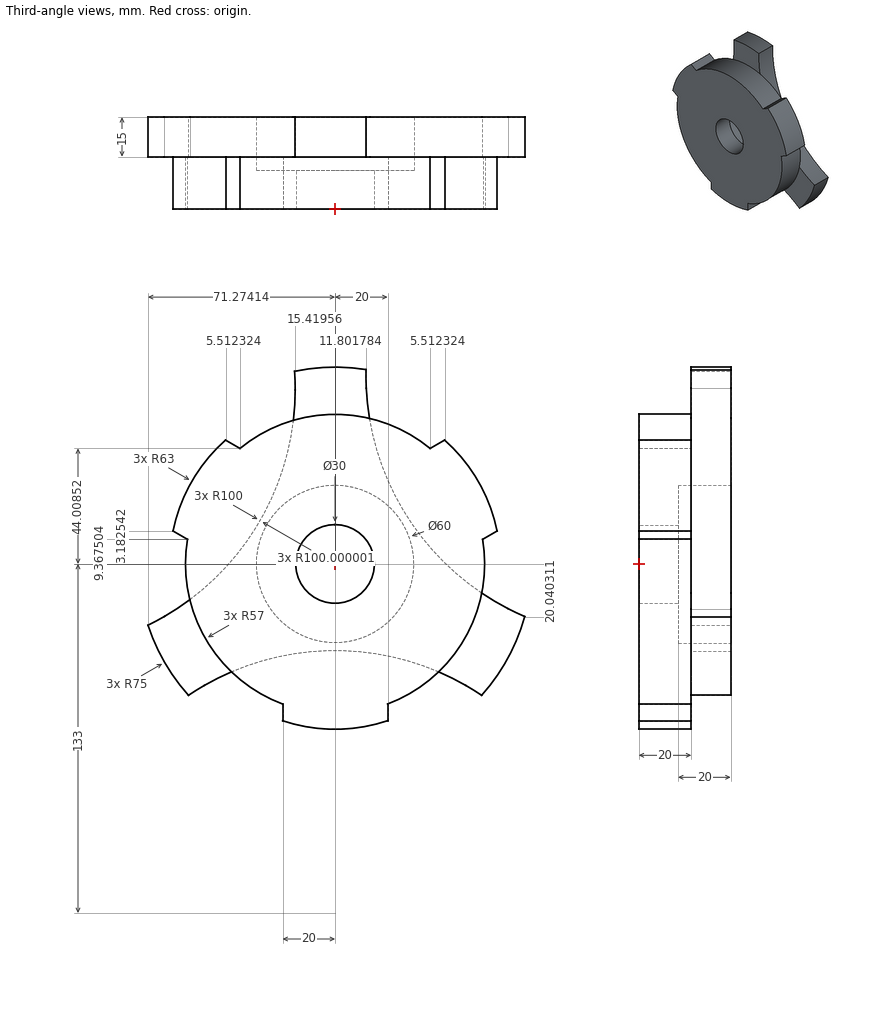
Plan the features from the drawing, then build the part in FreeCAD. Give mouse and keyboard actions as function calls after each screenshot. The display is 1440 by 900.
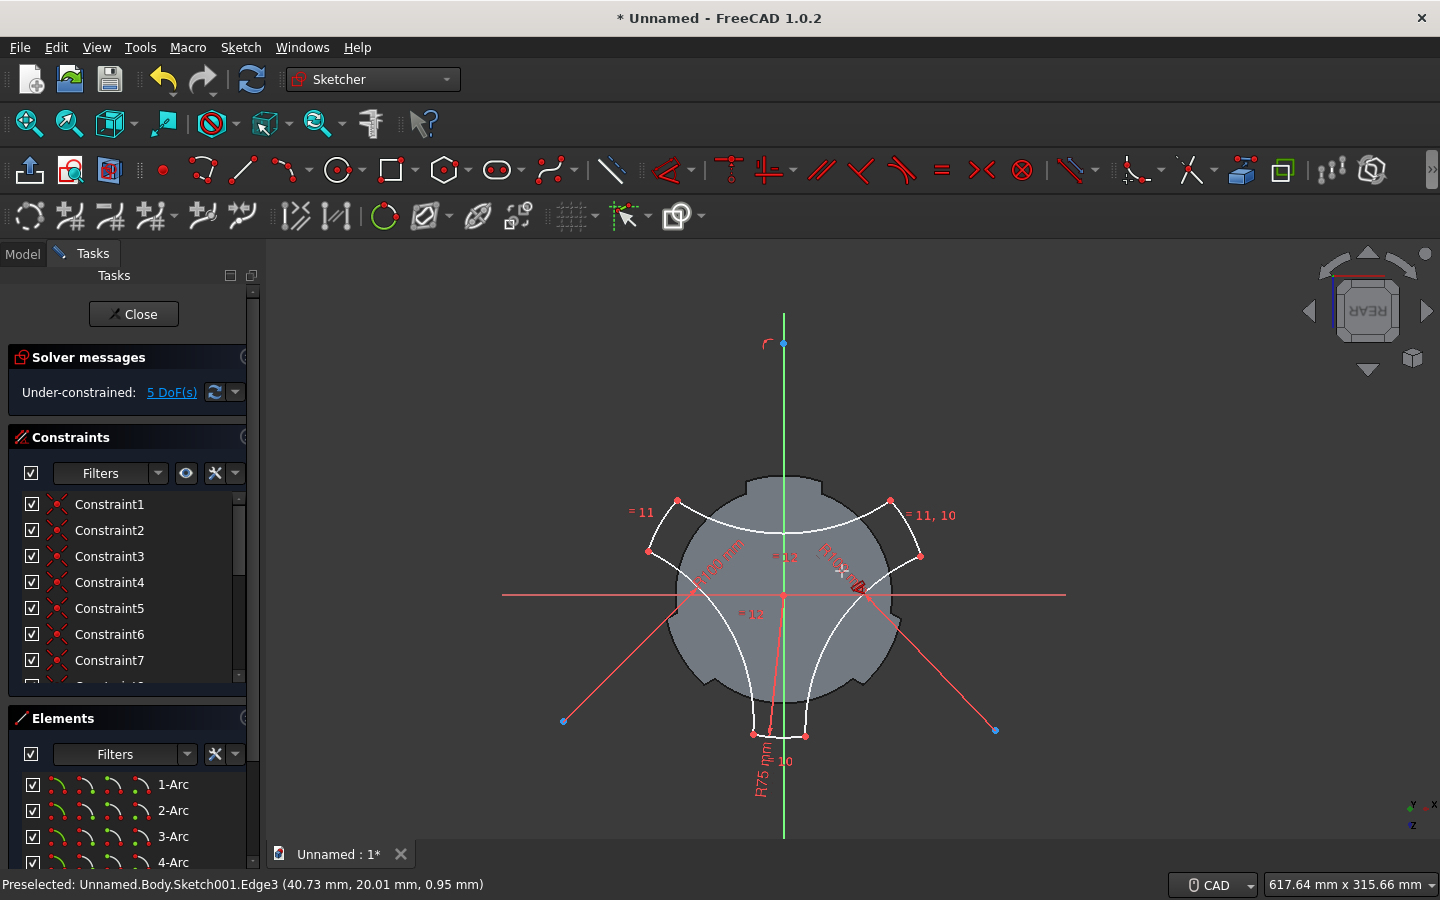
click(784, 343)
click(750, 469)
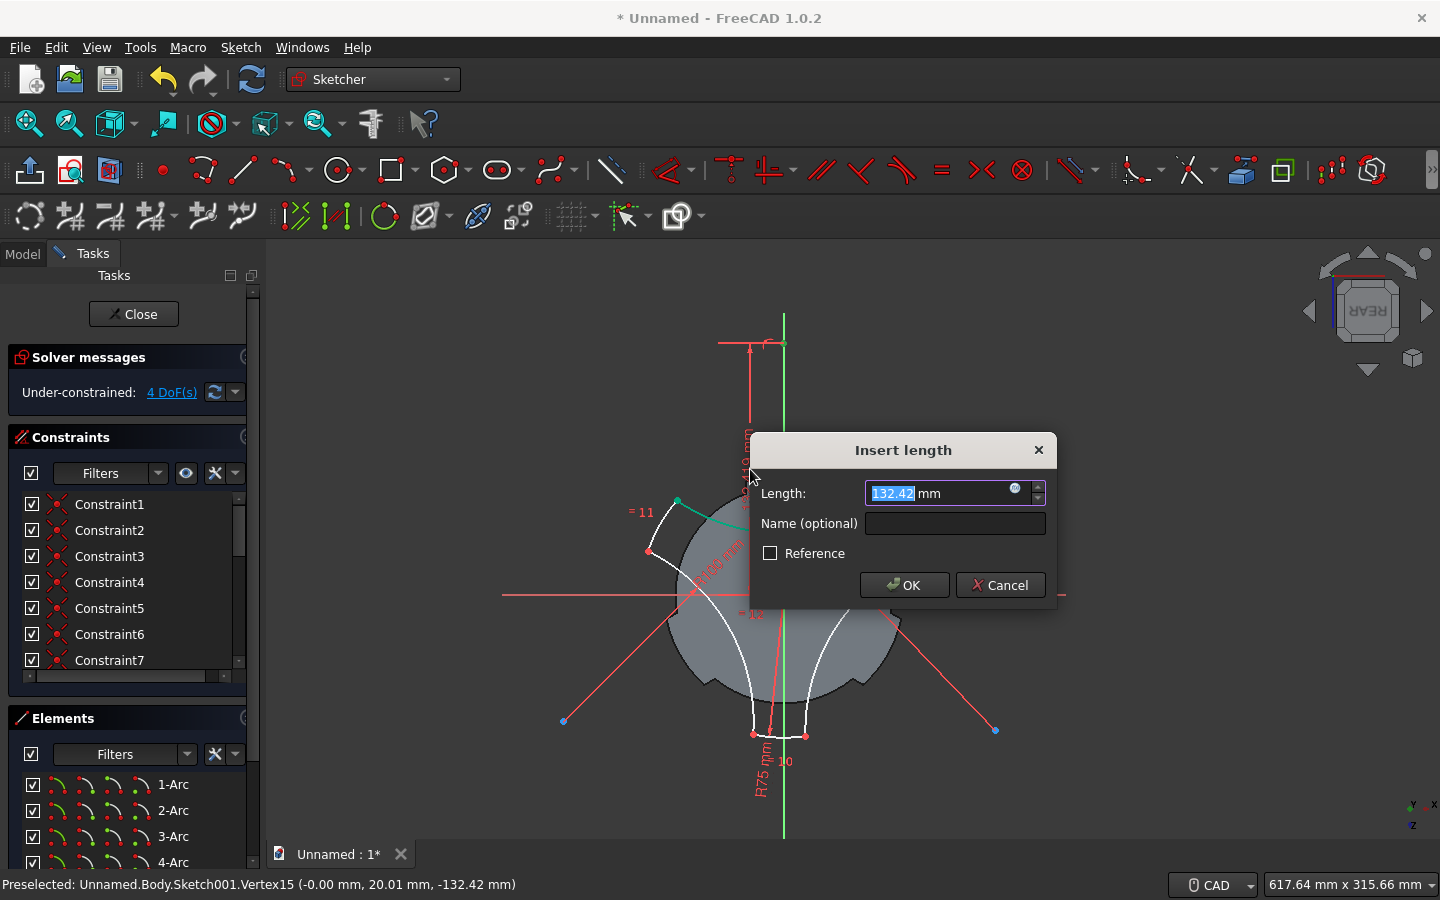
text(133)
key(Return)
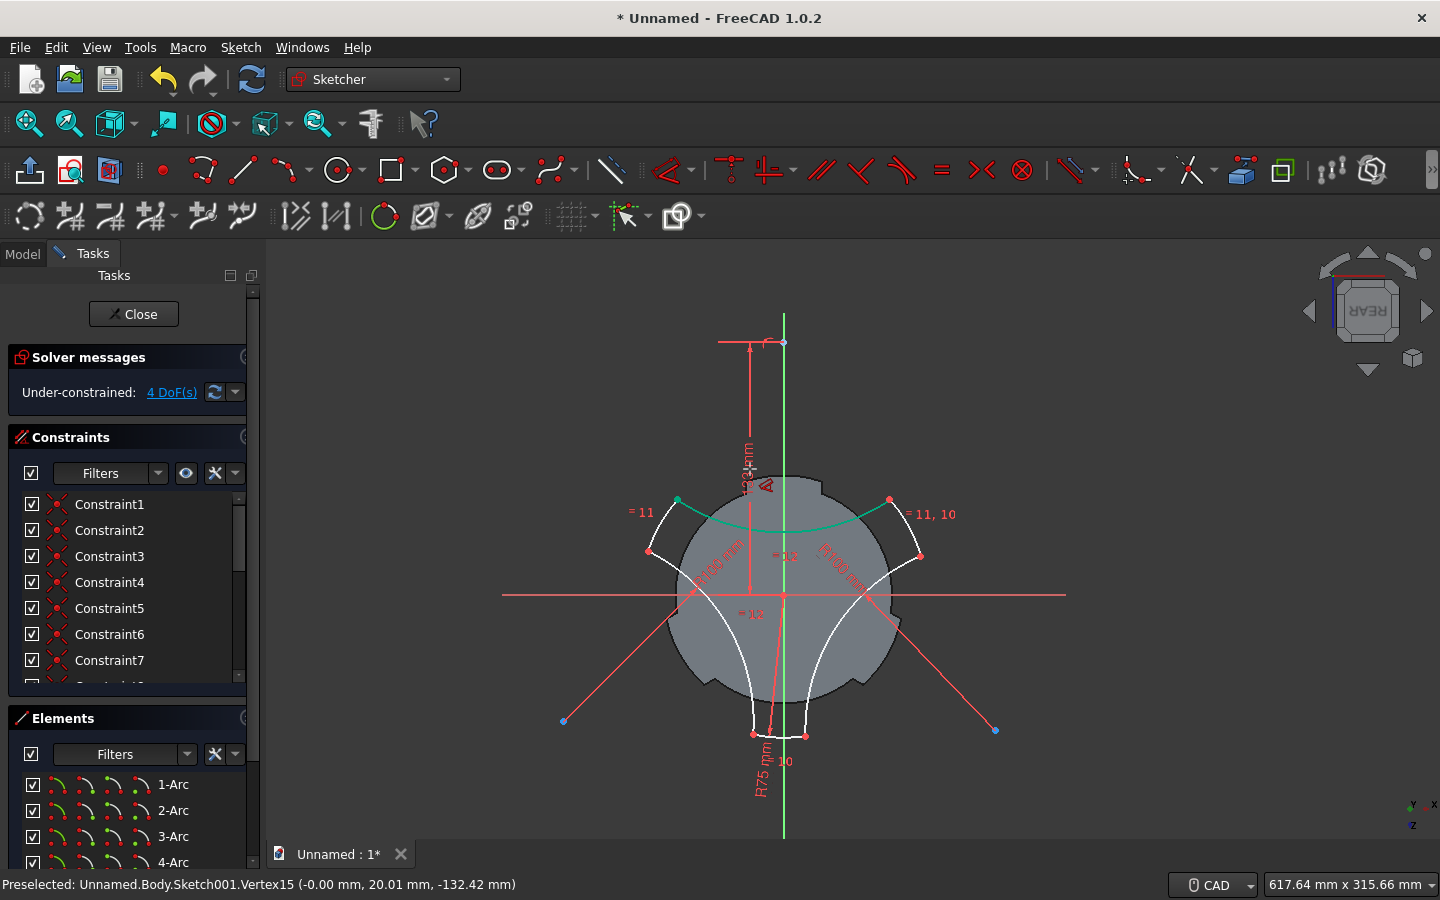
scroll(753, 734, up, 2)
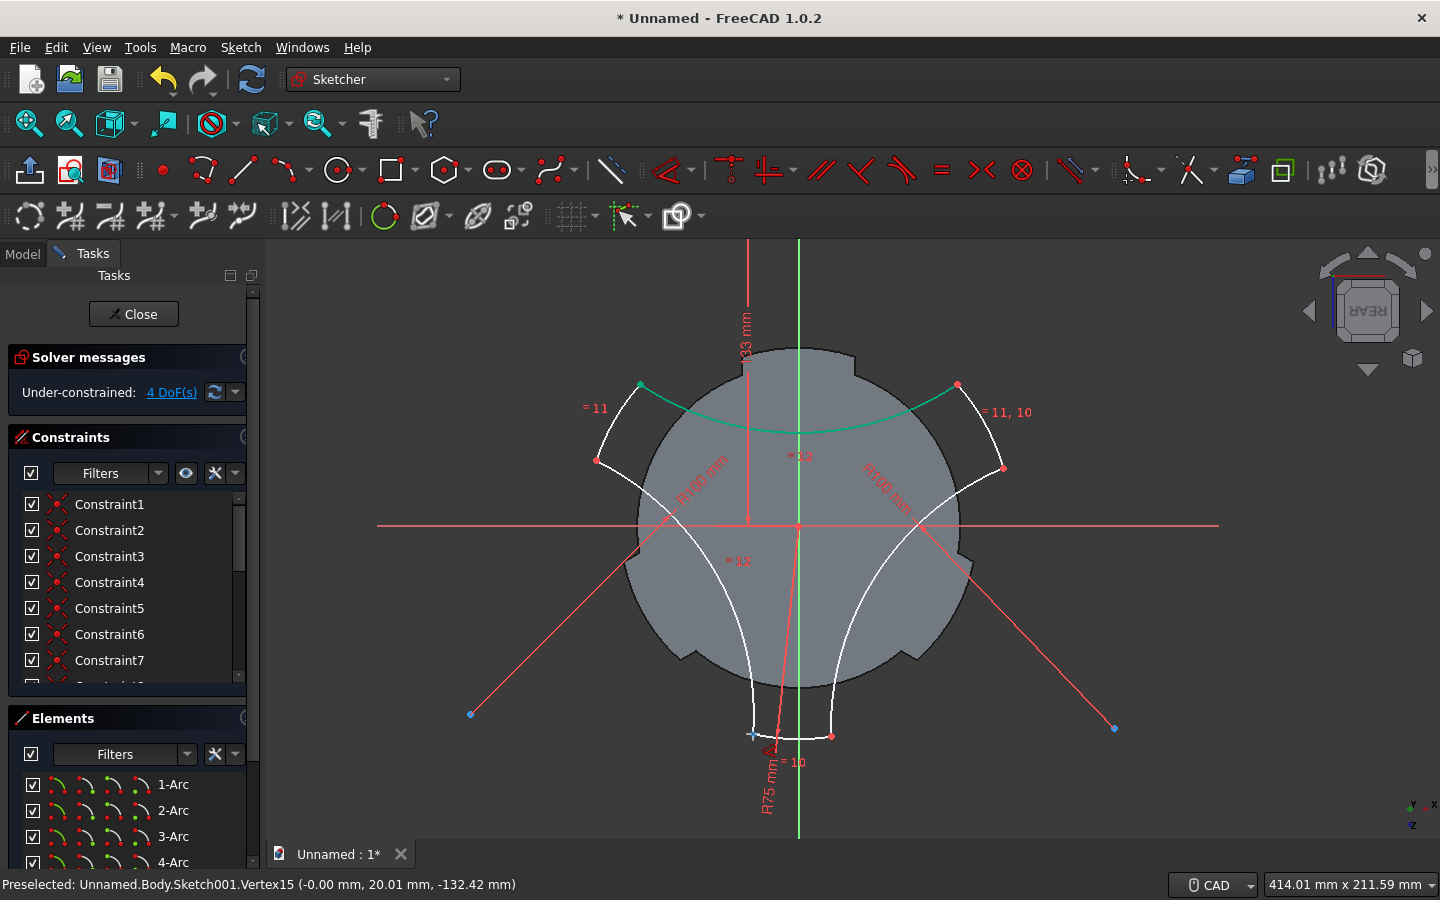
click(753, 734)
click(776, 492)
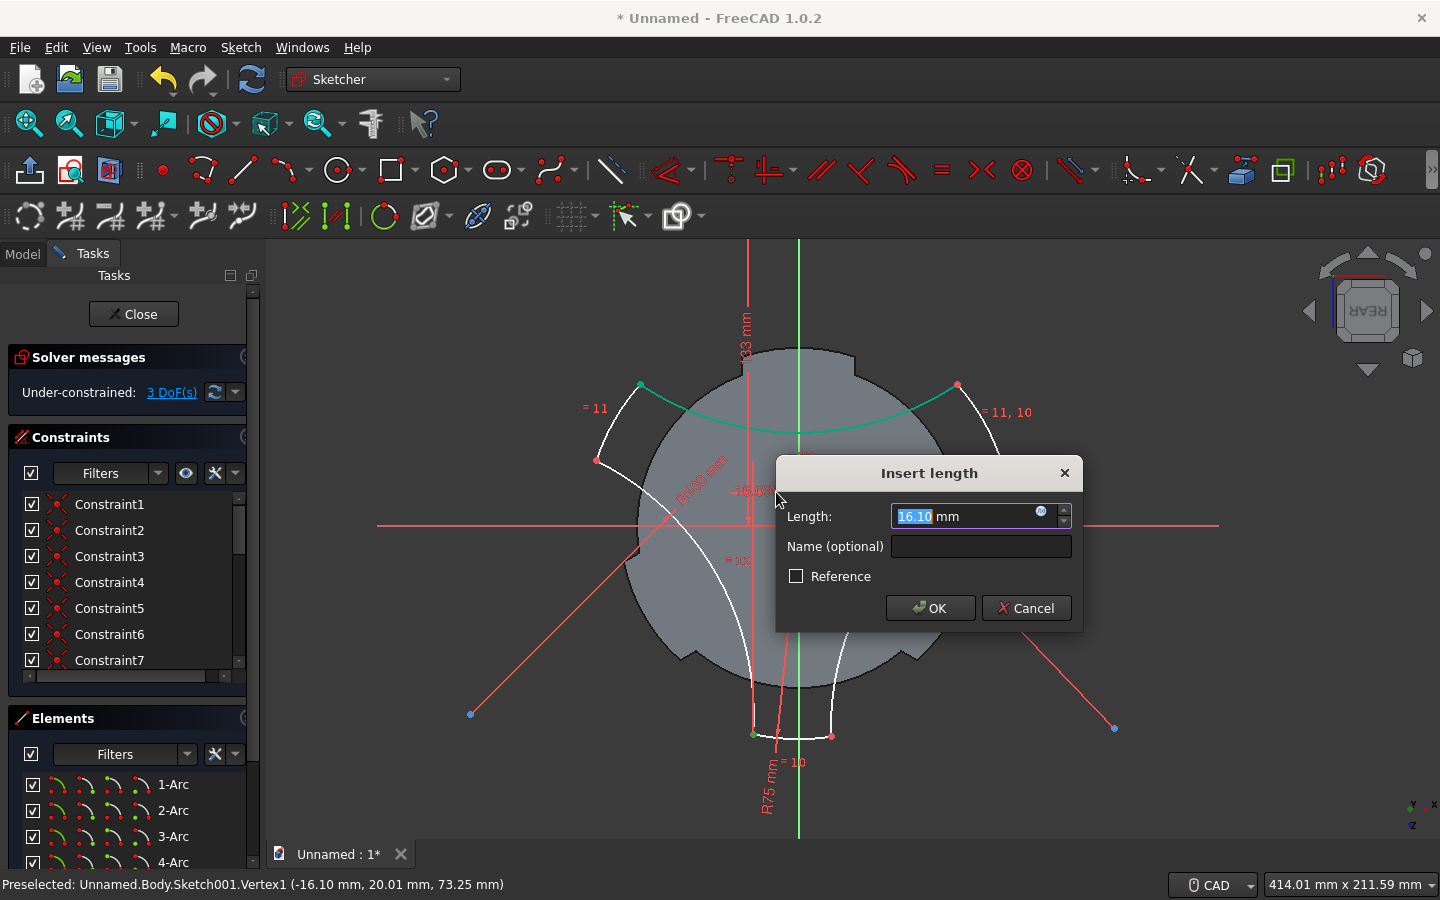
text(15.41956)
key(Return)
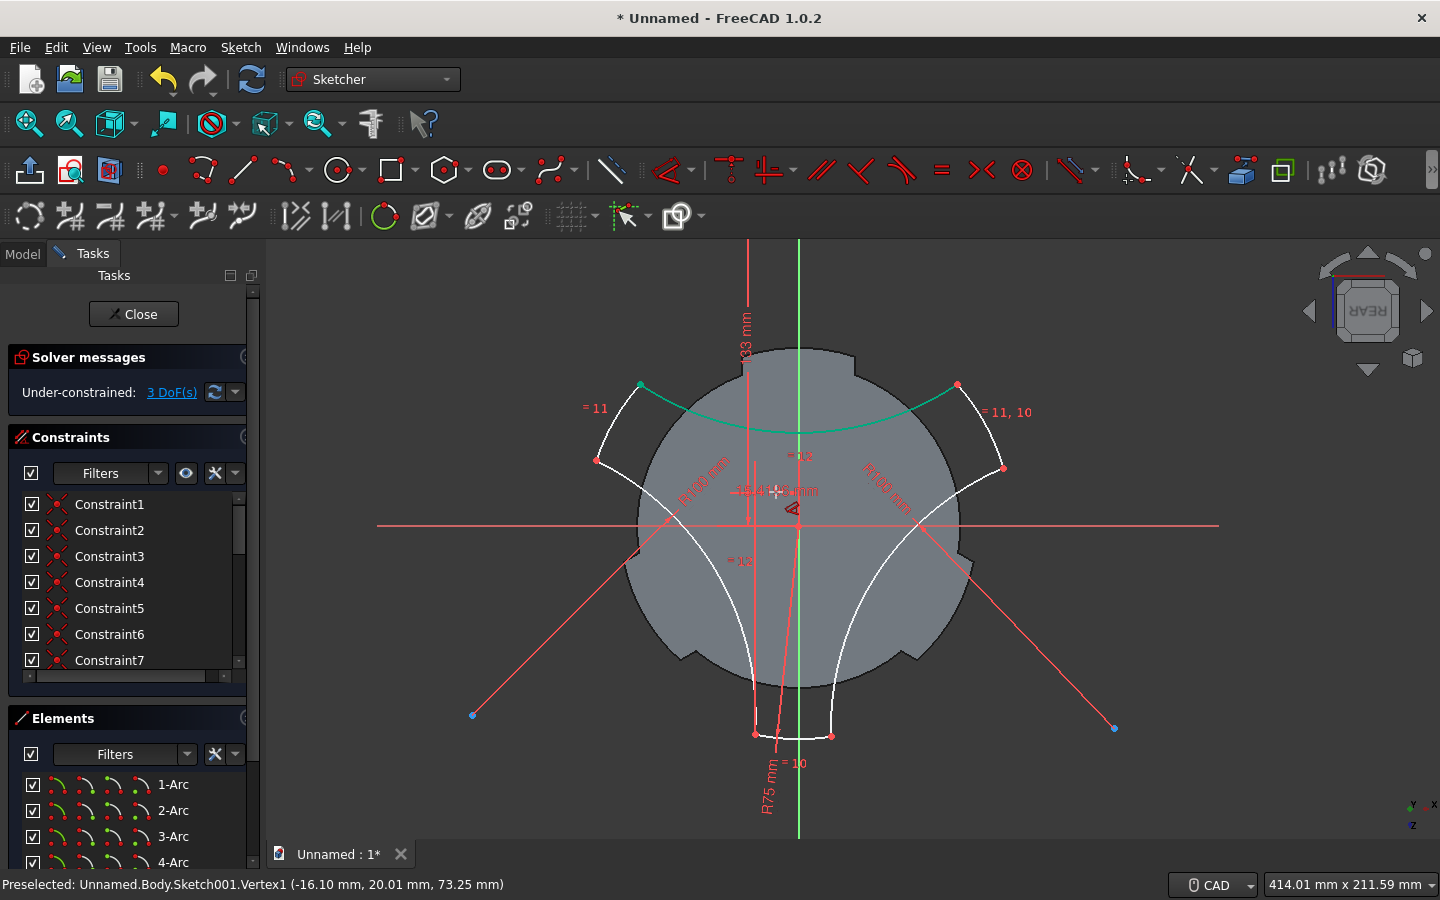
click(596, 461)
click(651, 427)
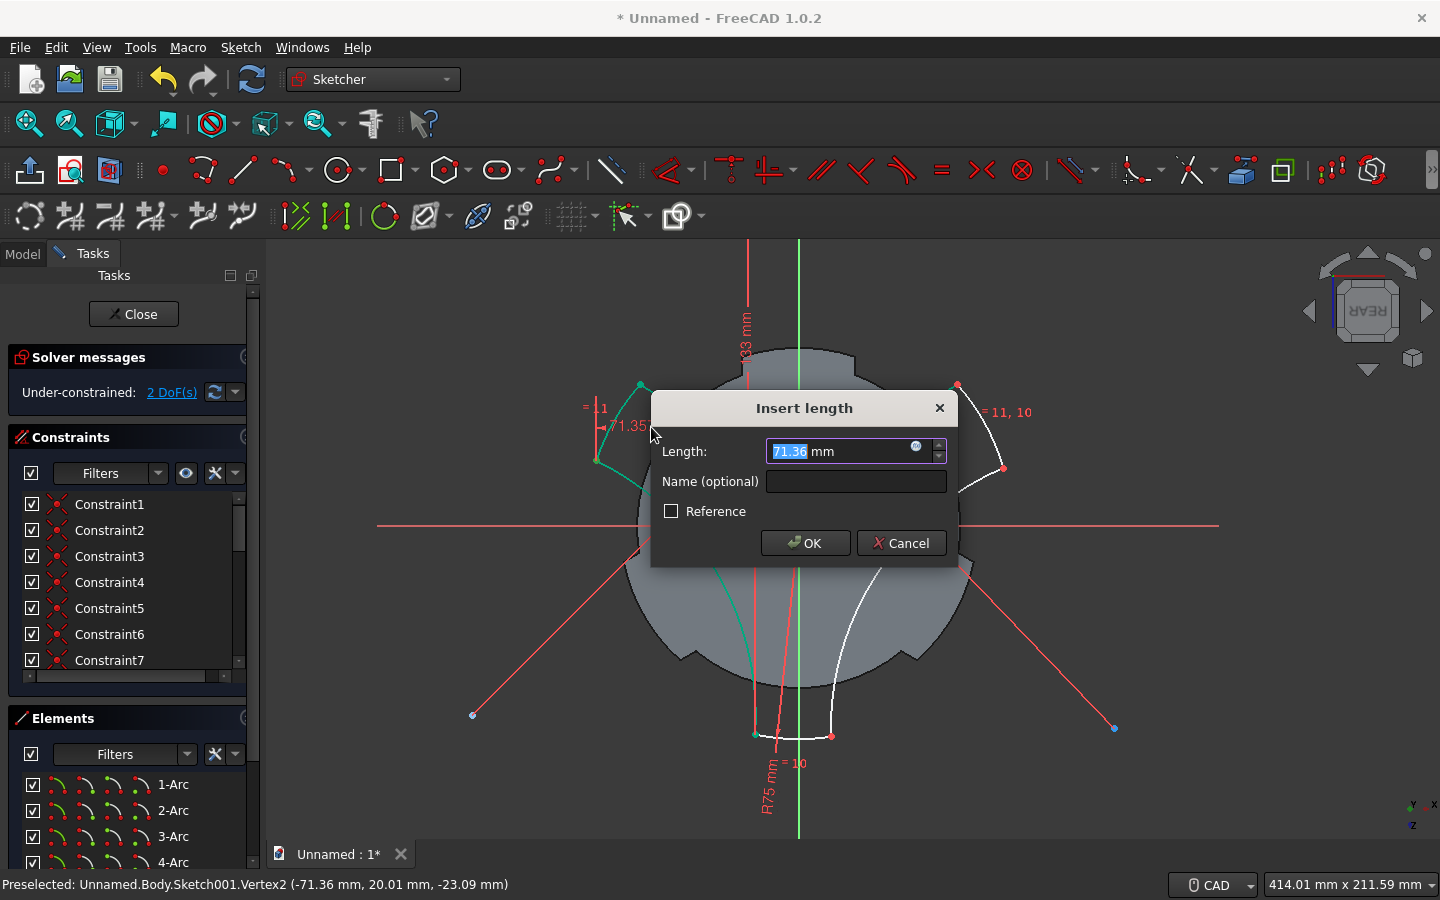
text(71.27414)
key(Return)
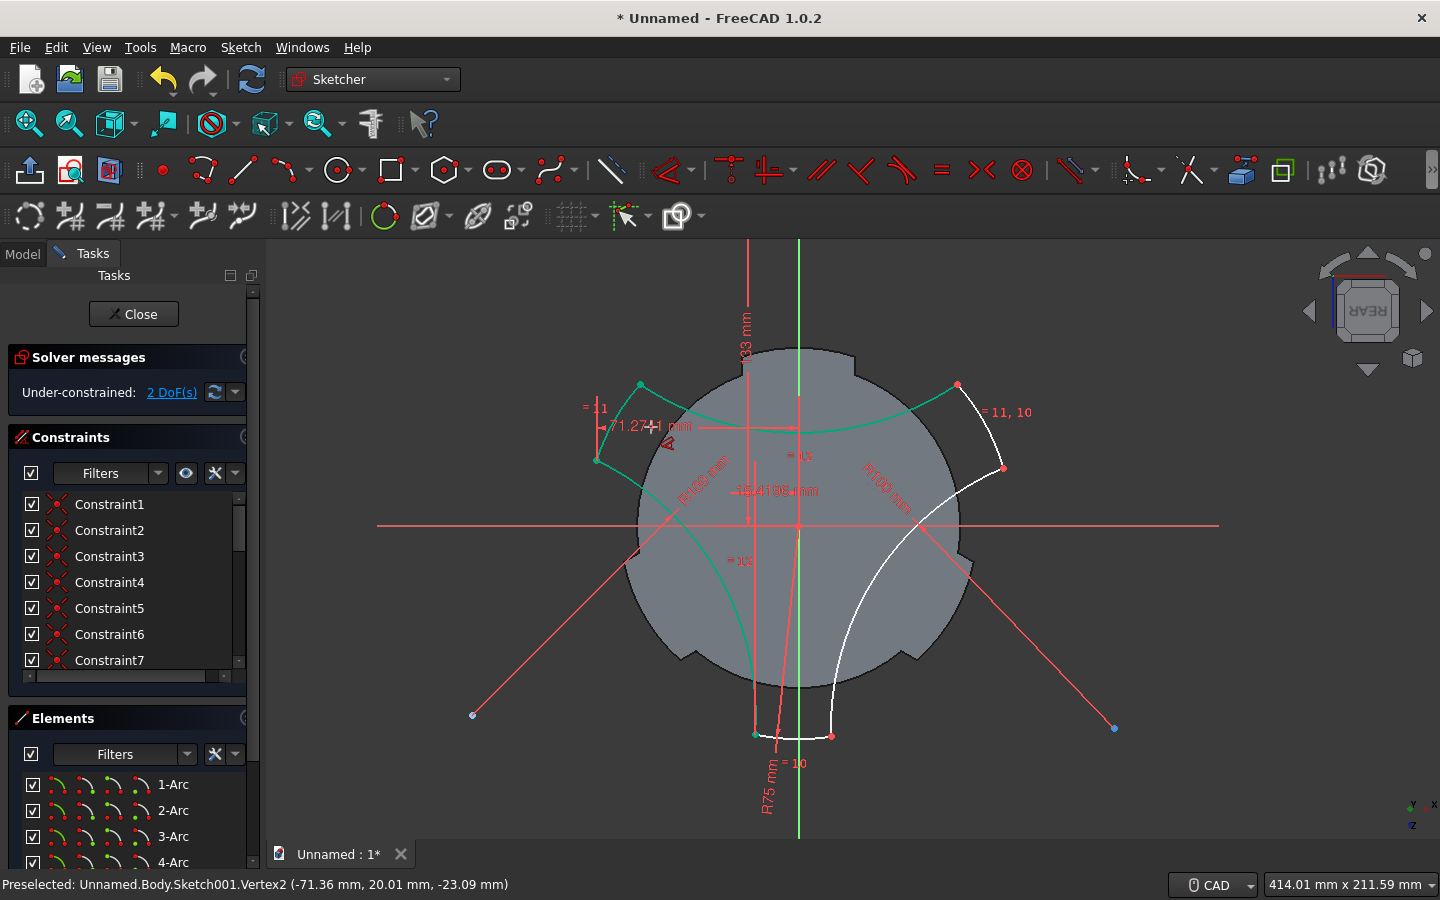
click(831, 737)
click(815, 468)